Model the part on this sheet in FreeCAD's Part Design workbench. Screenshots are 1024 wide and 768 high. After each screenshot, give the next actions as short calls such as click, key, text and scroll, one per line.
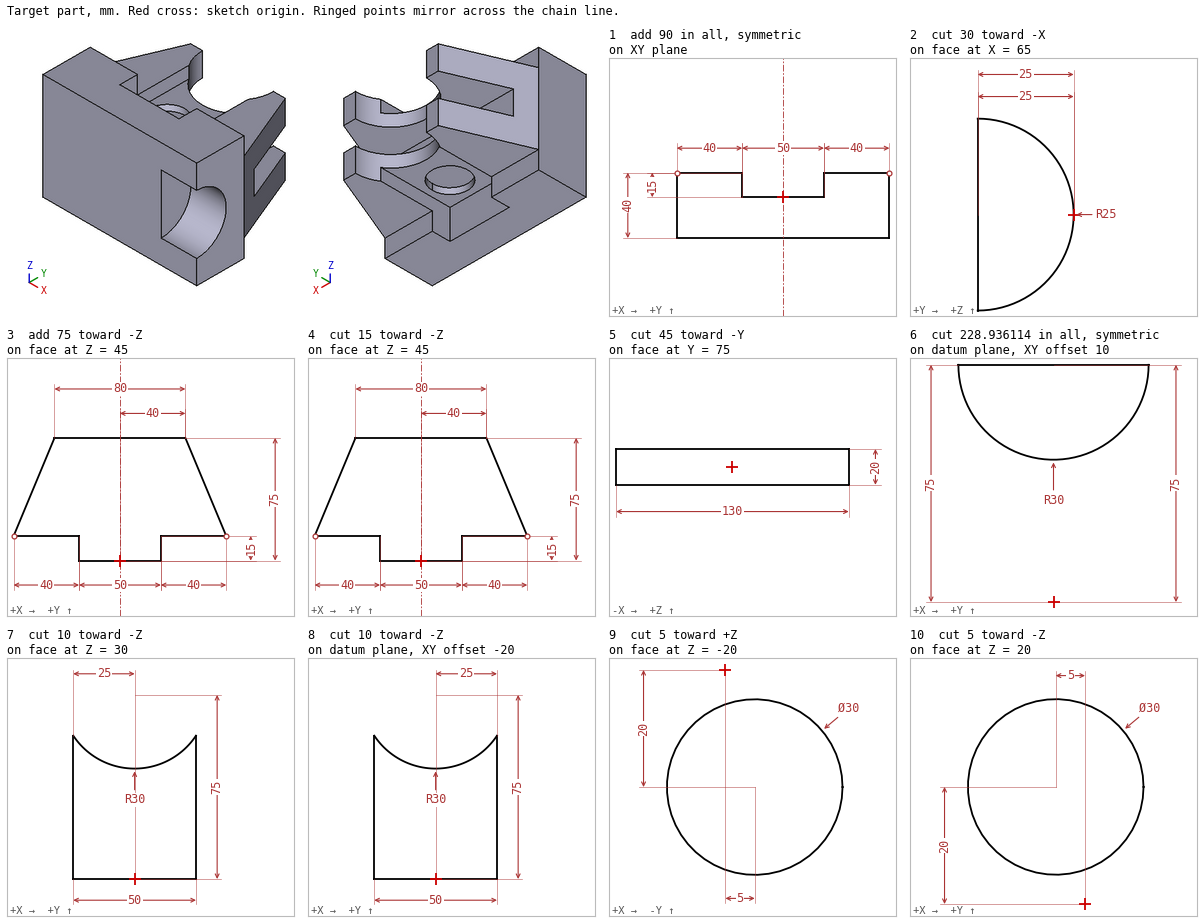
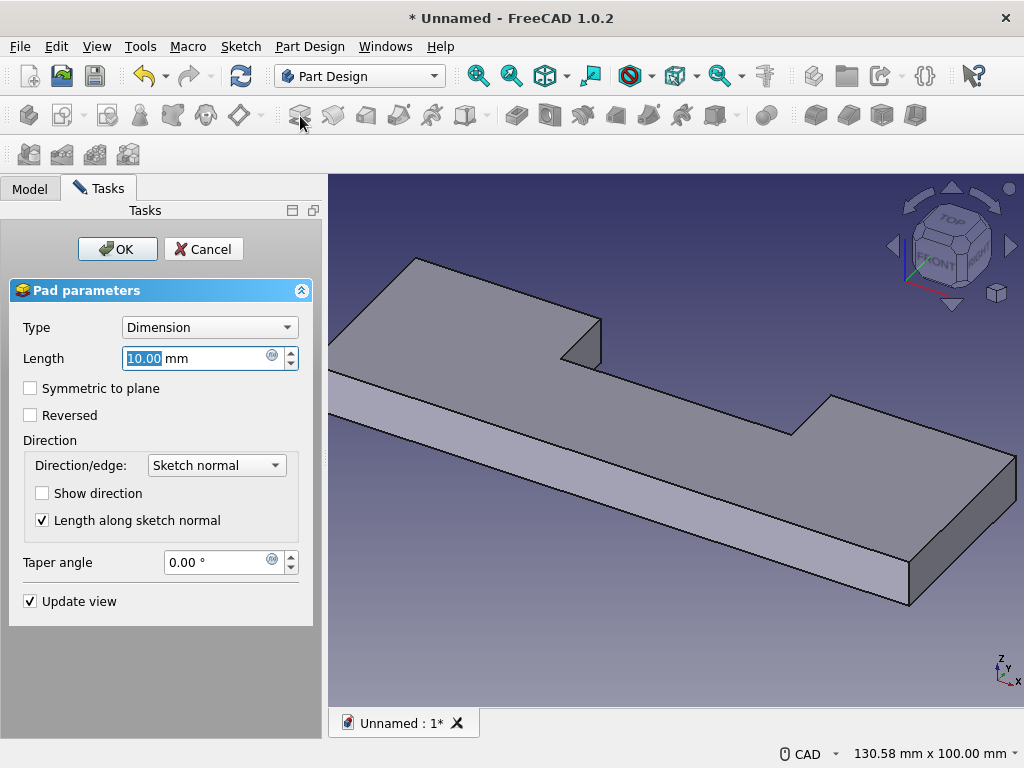
text(90)
key(Tab)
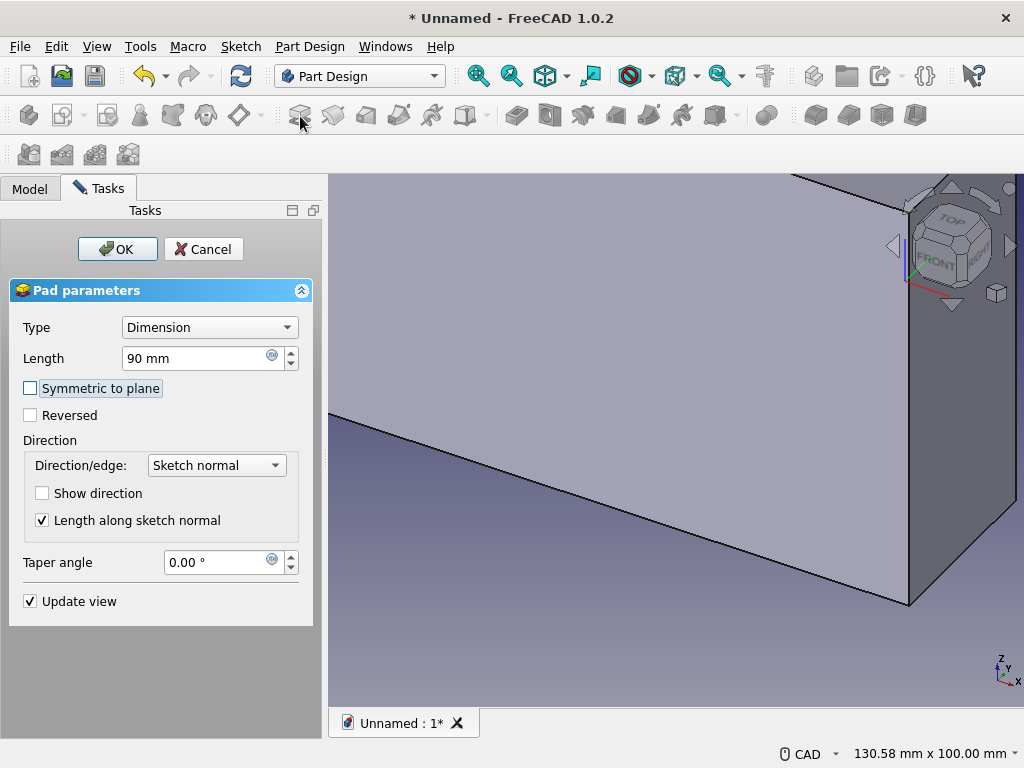
click(31, 388)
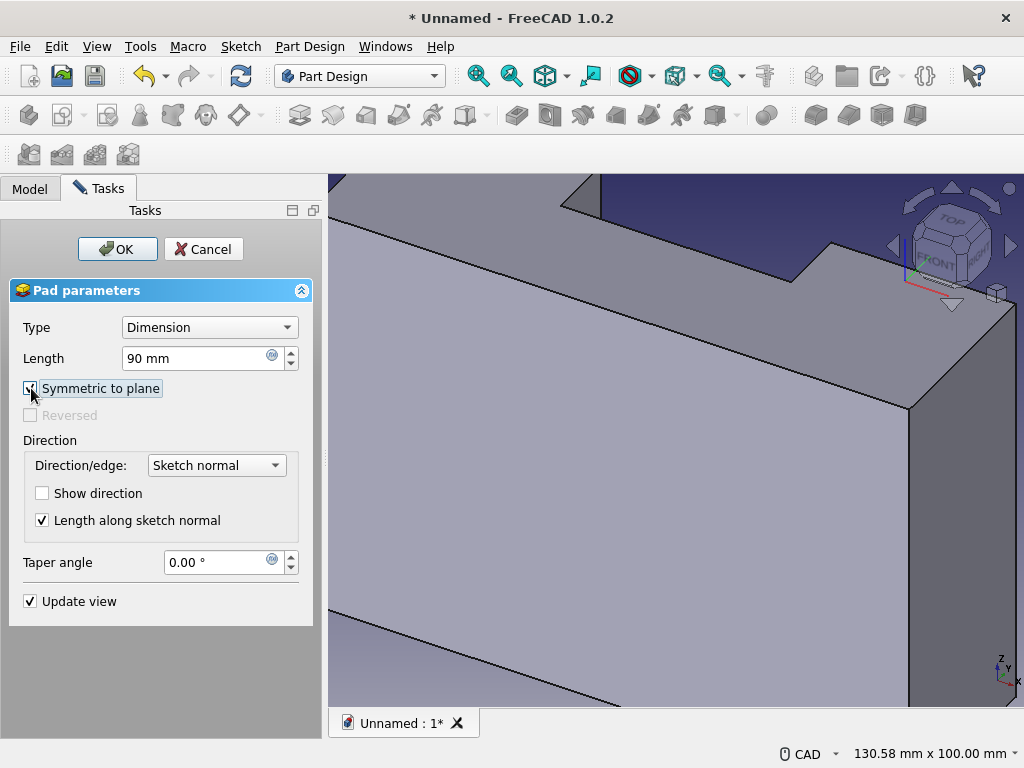
click(118, 249)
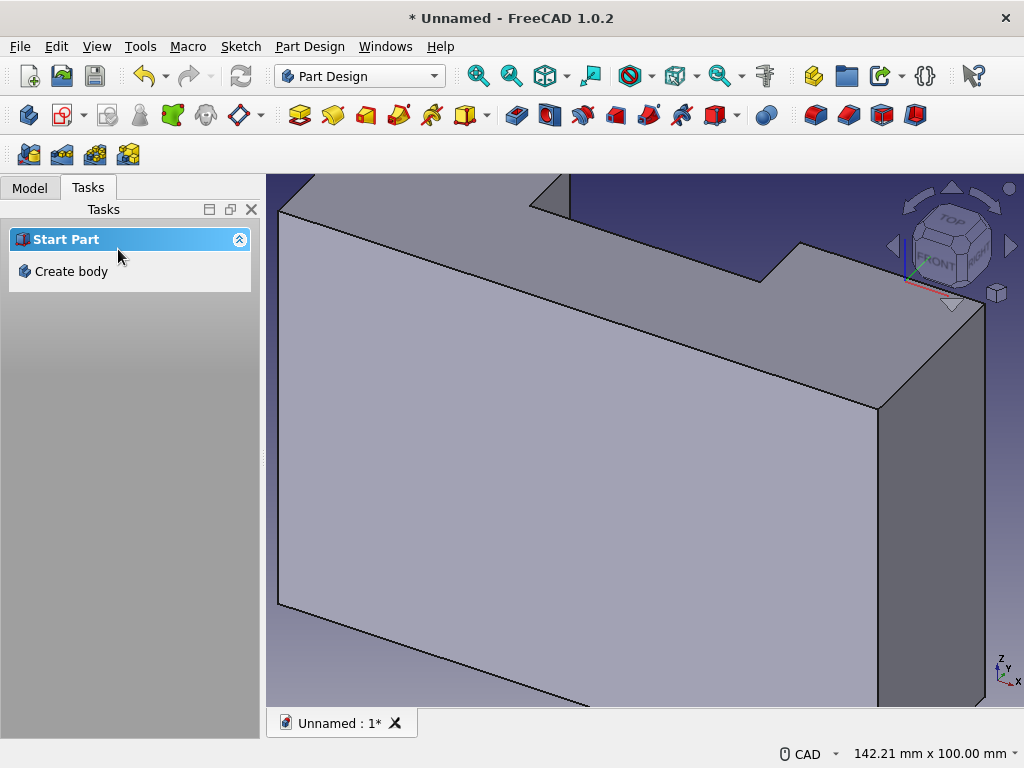
key(v)
key(f)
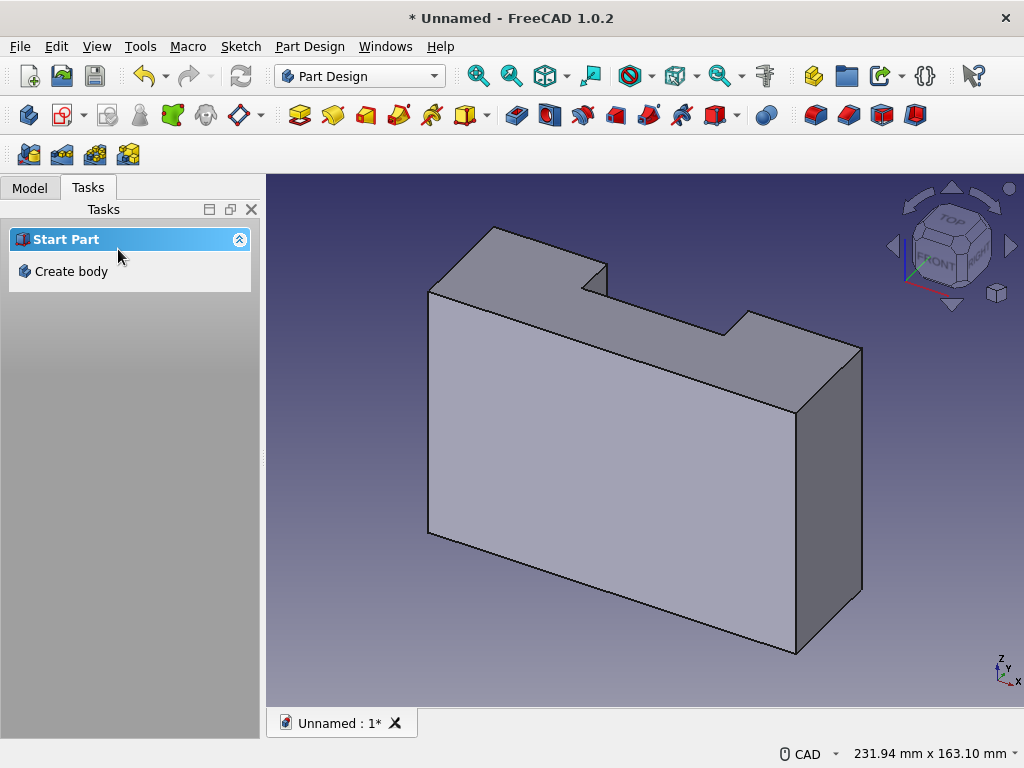
click(829, 466)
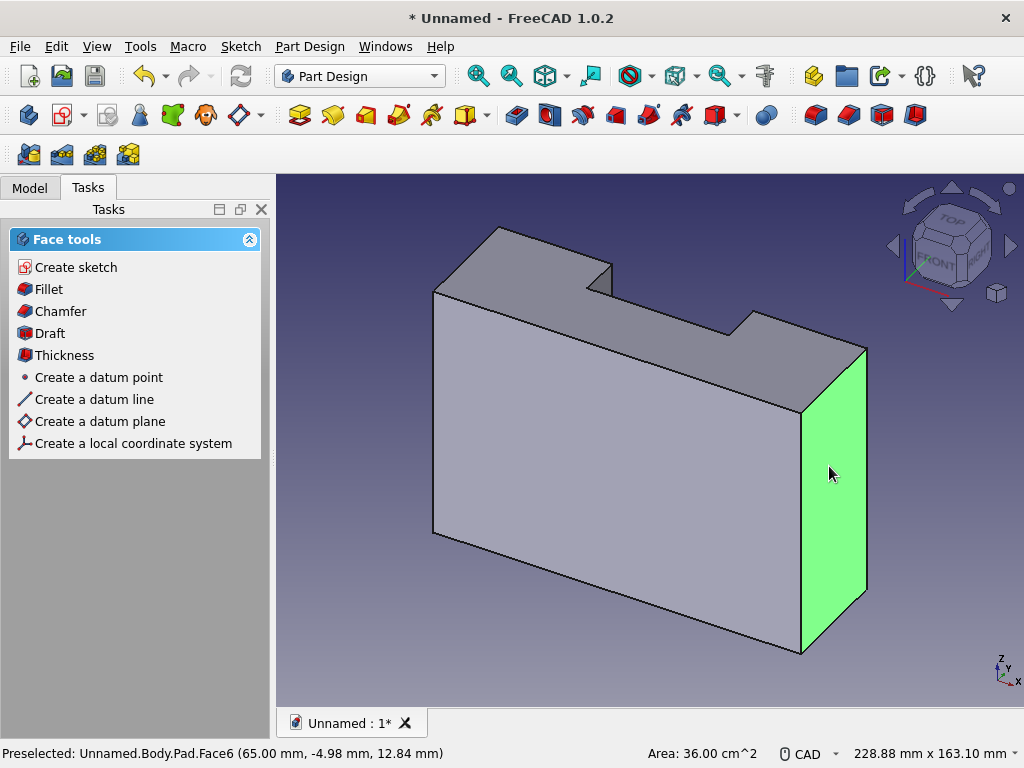
click(62, 116)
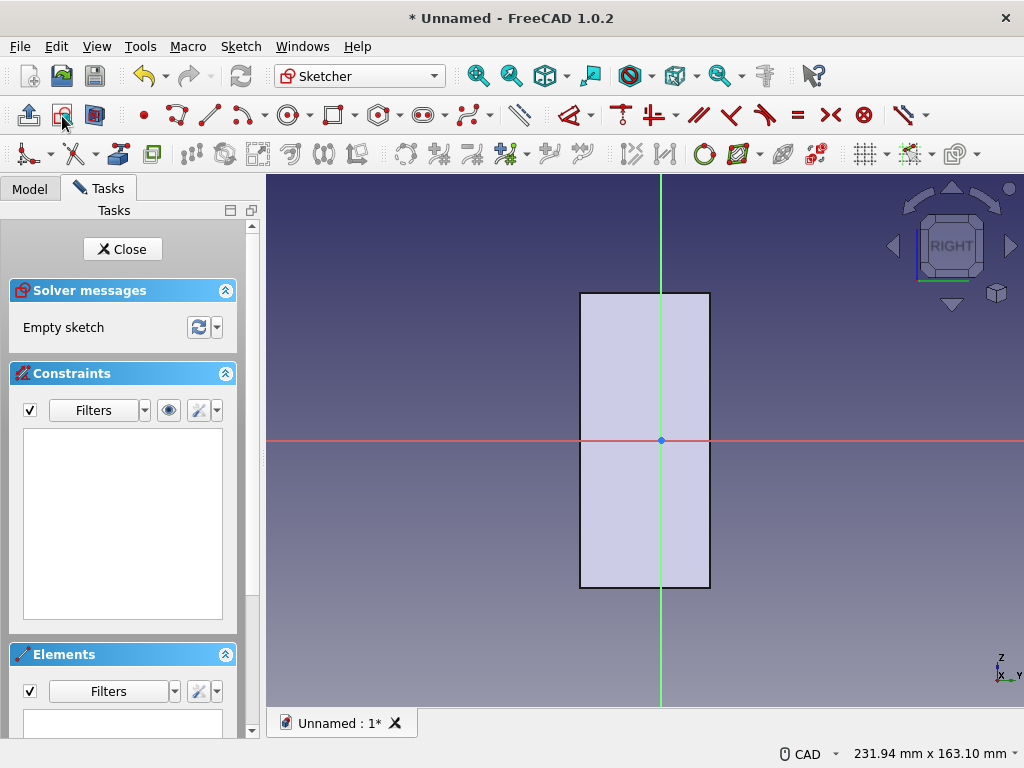
scroll(656, 440, up, 4)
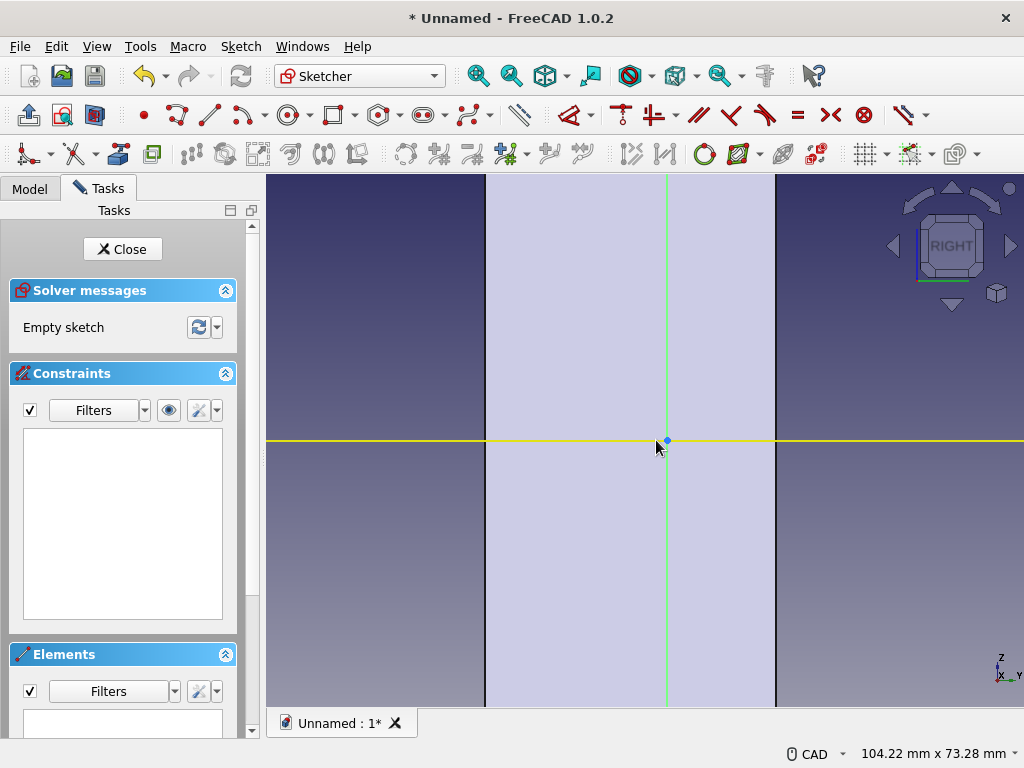
key(g)
key(l)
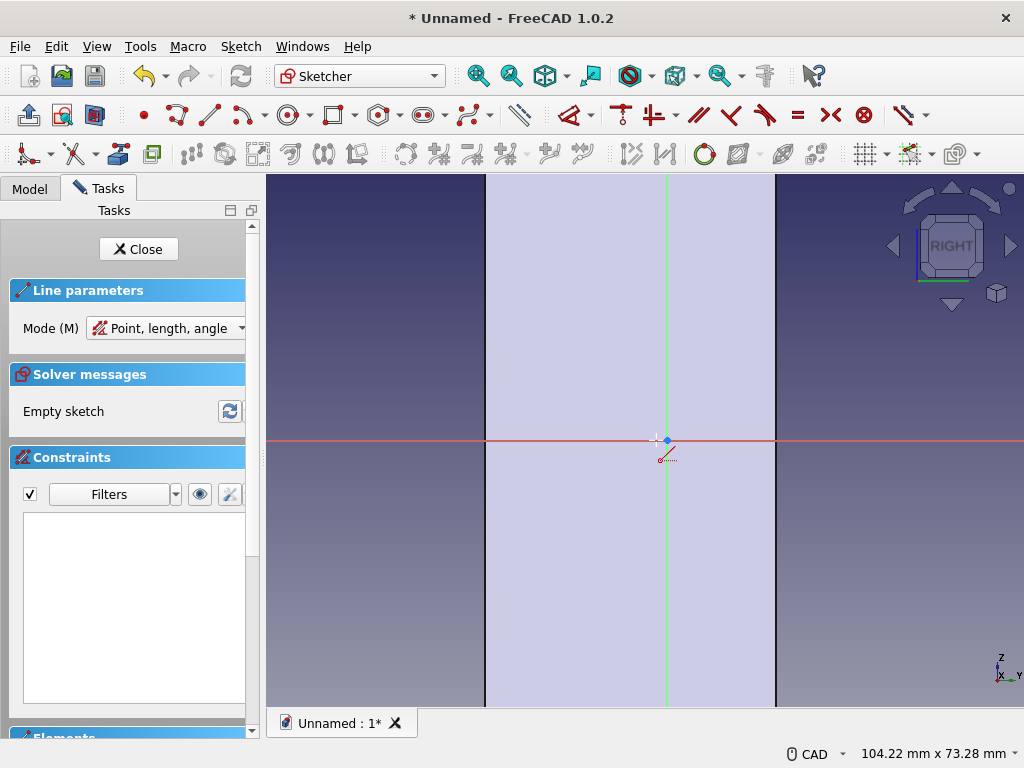
click(485, 259)
click(485, 622)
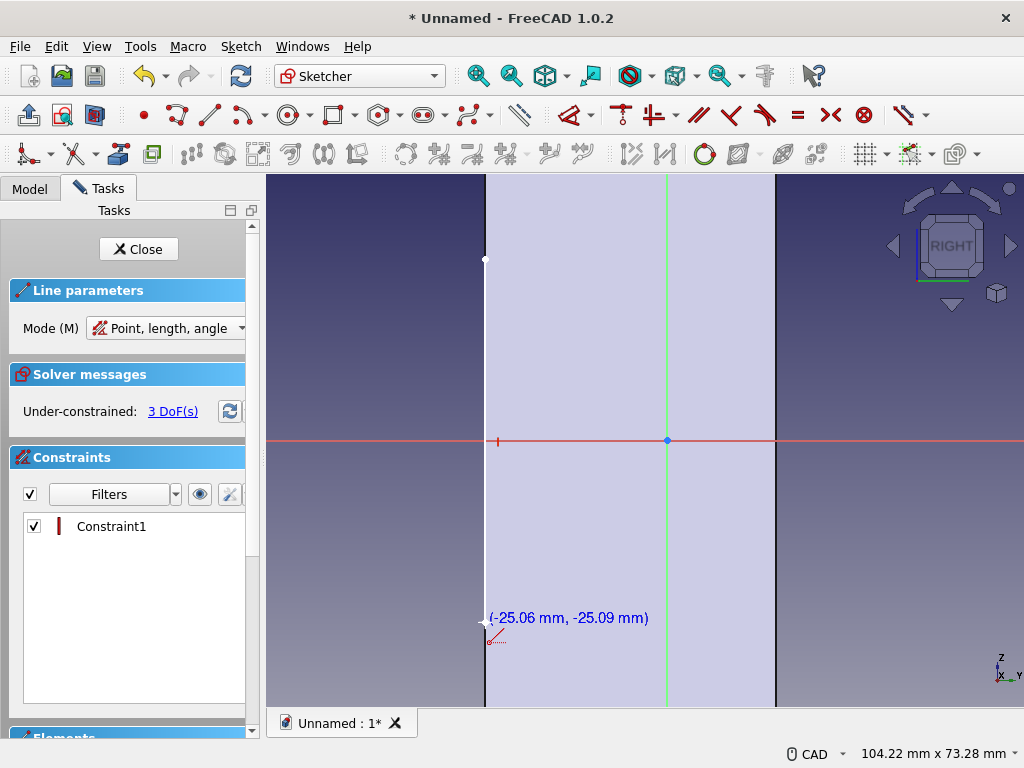
key(g)
key(3)
key(a)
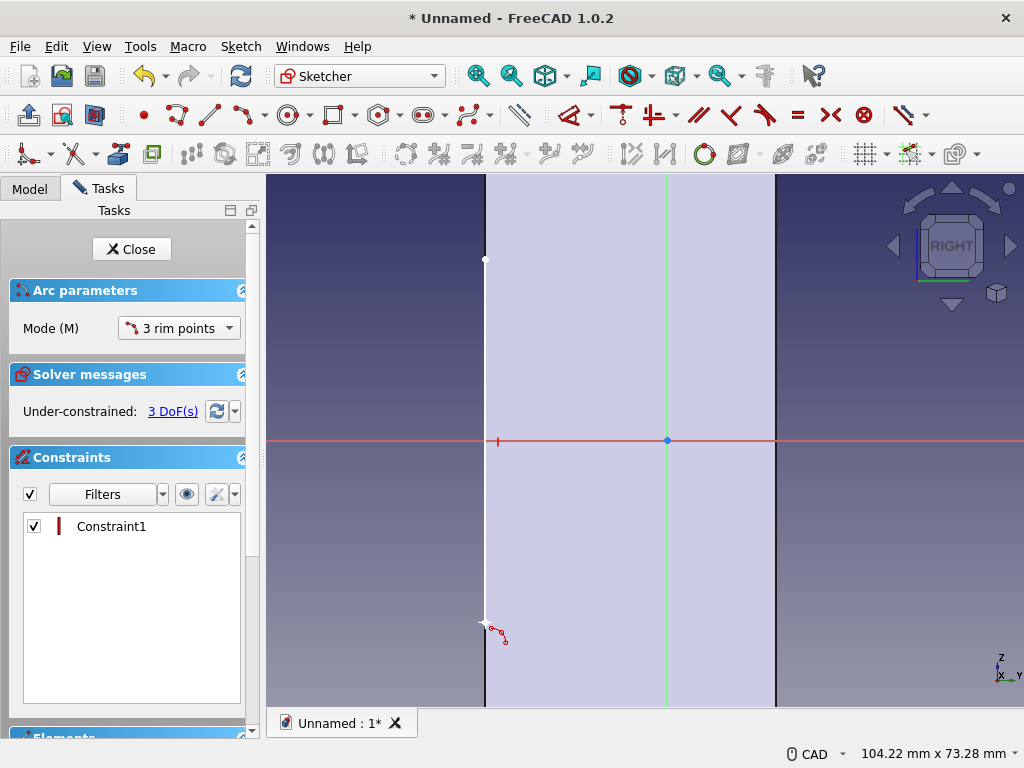
click(485, 623)
click(485, 260)
click(633, 547)
key(Escape)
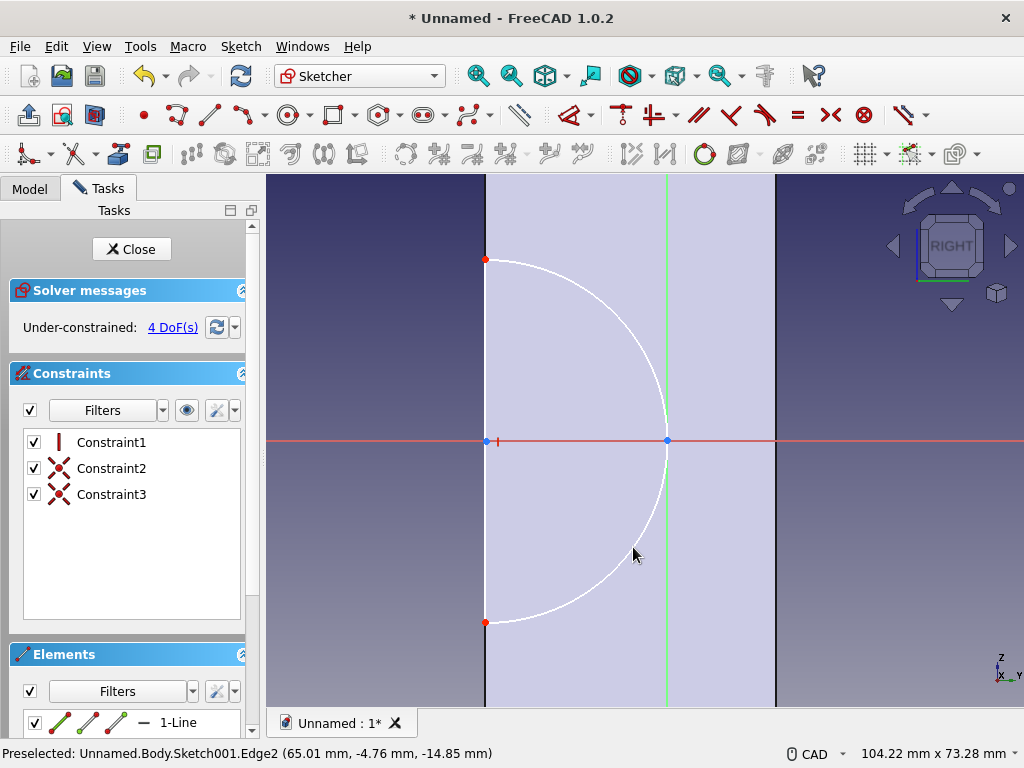
click(486, 441)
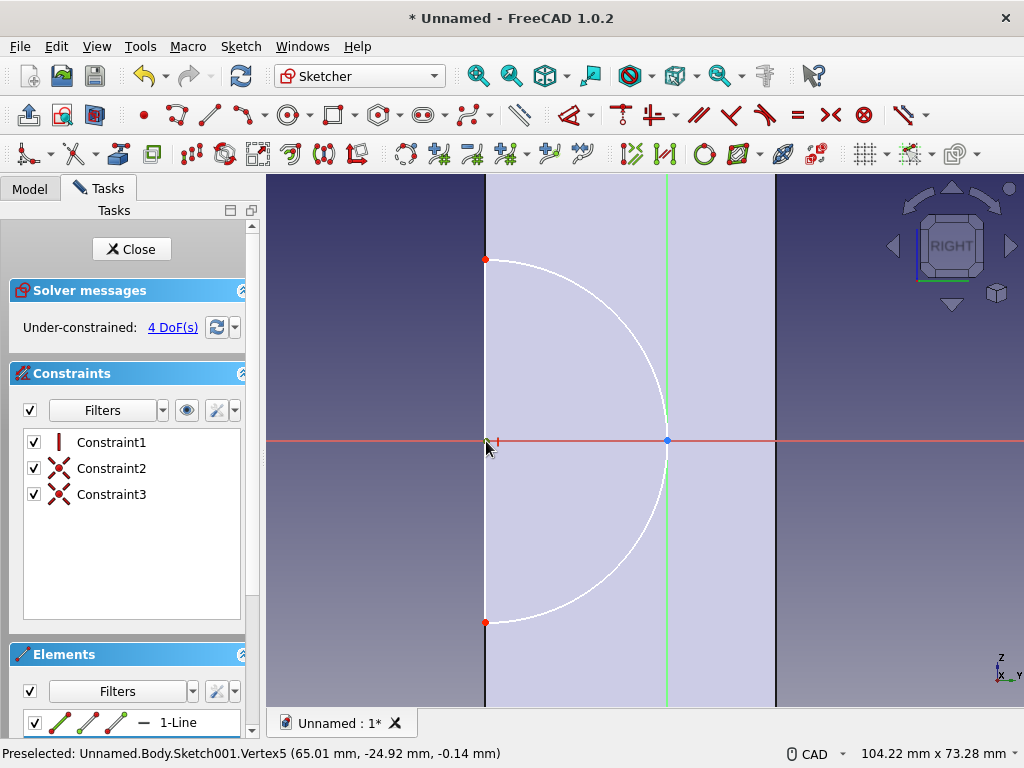
click(334, 440)